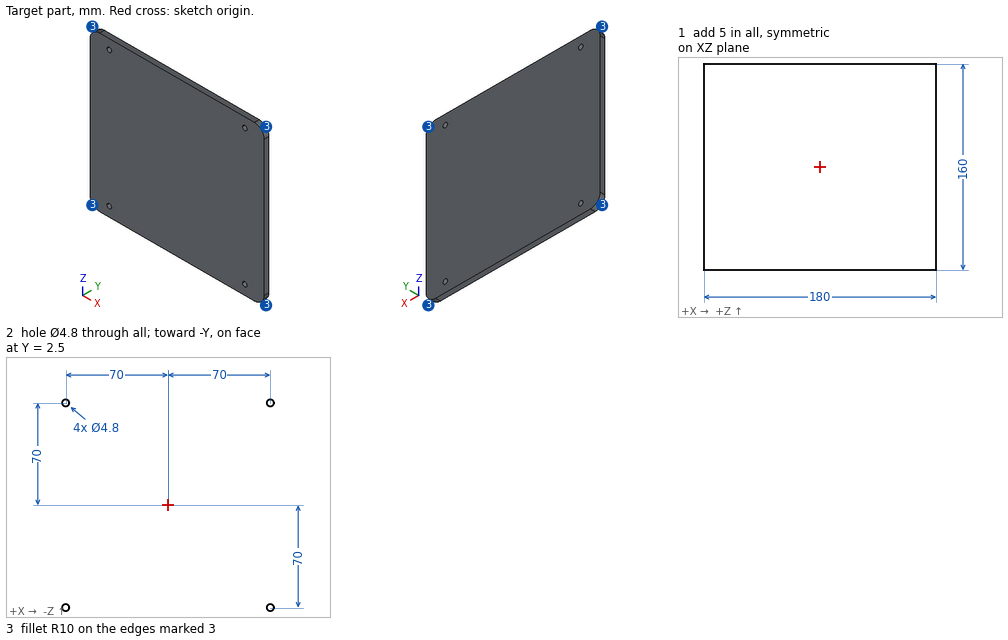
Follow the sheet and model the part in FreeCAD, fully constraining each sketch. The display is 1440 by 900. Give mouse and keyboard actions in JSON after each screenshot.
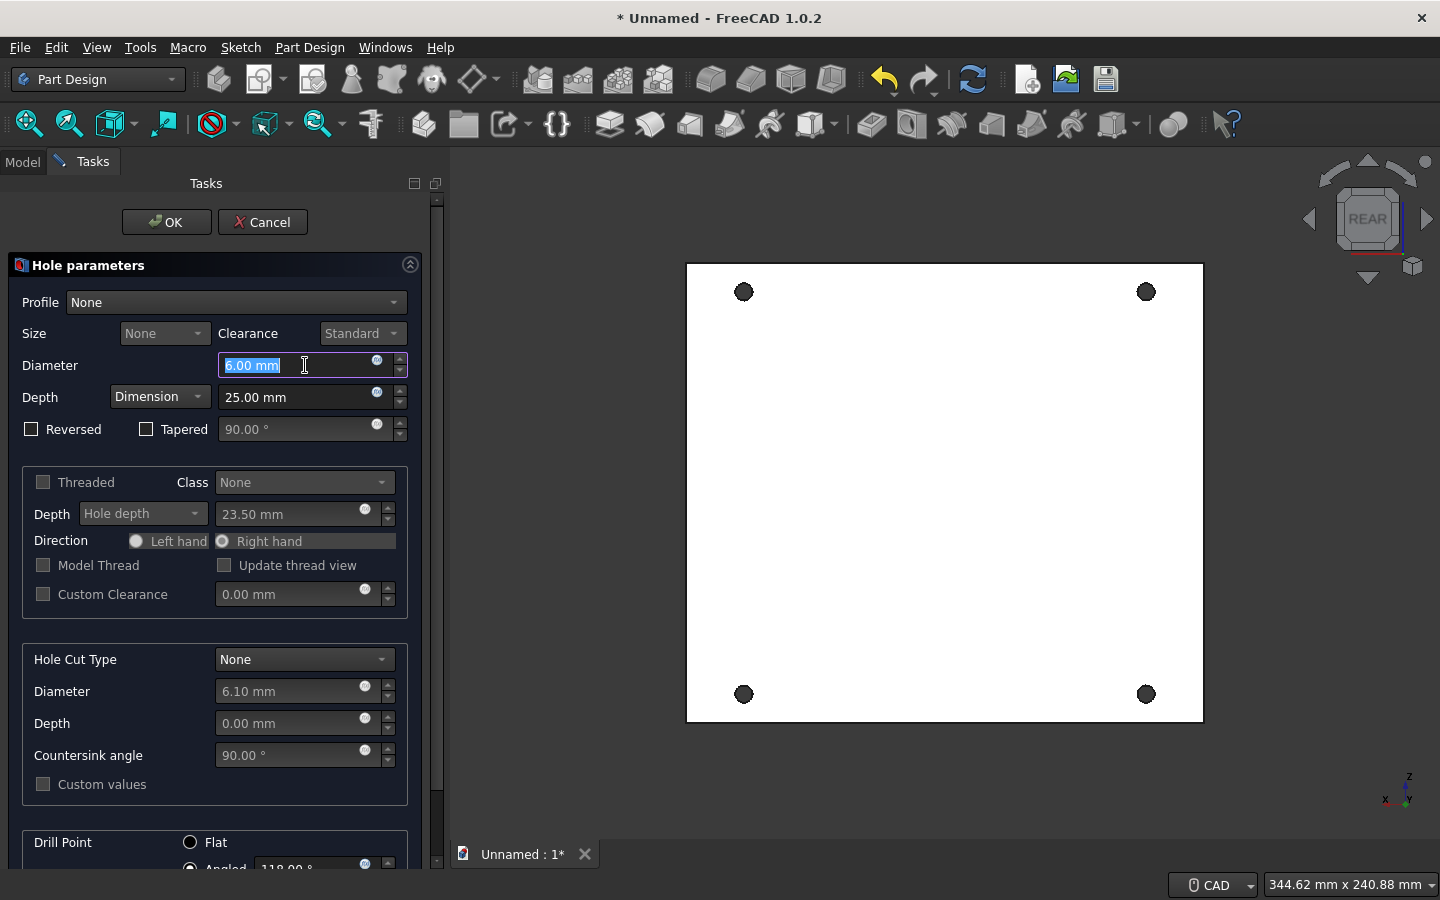
{"action": "type", "text": "4.8"}
{"action": "key", "text": "Tab"}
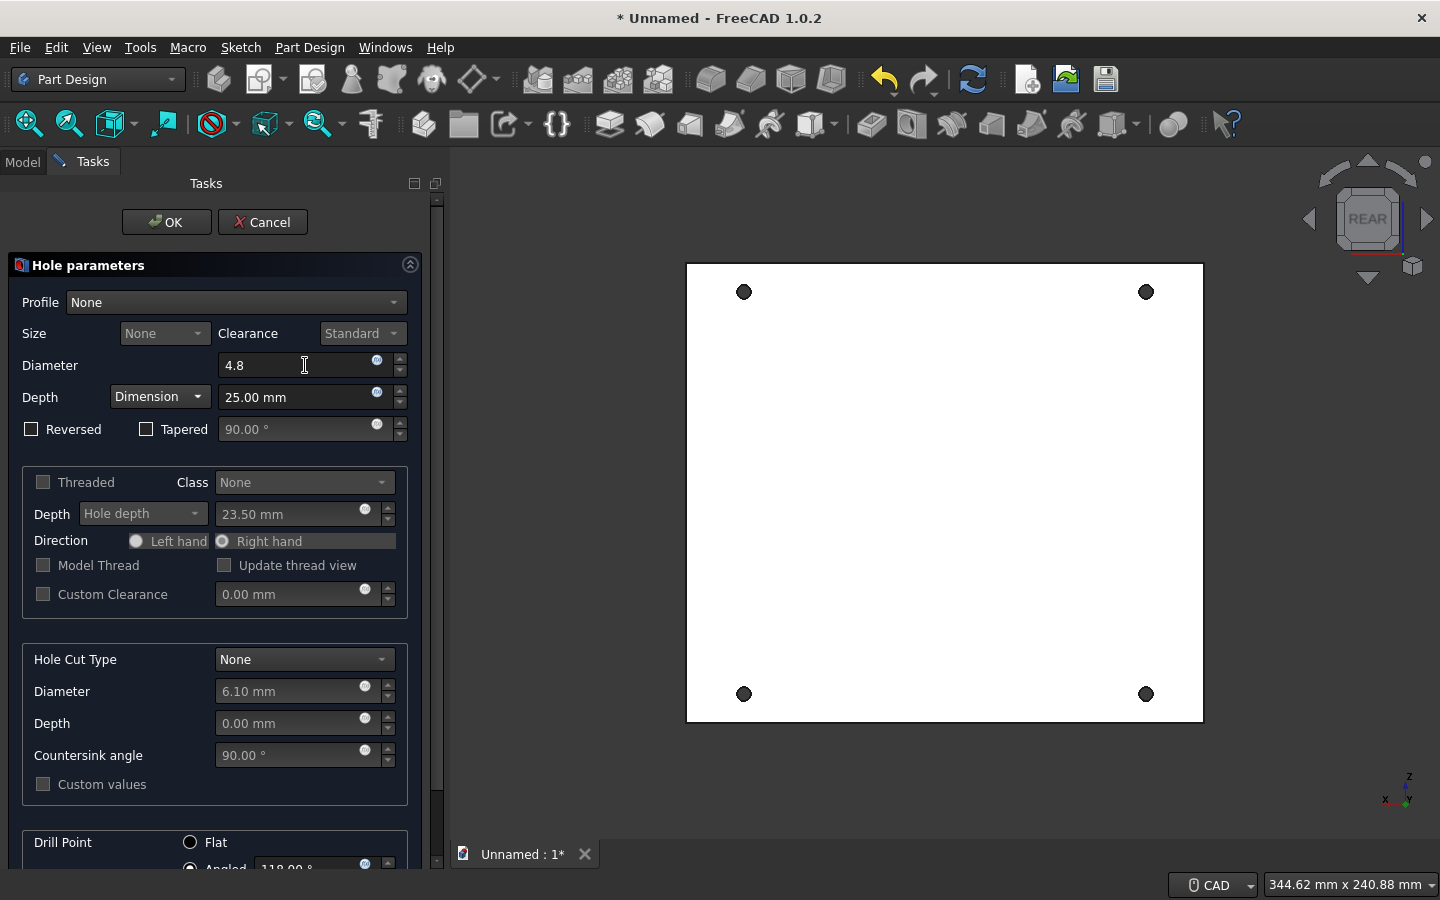
{"action": "left_click", "coordinate": [161, 396]}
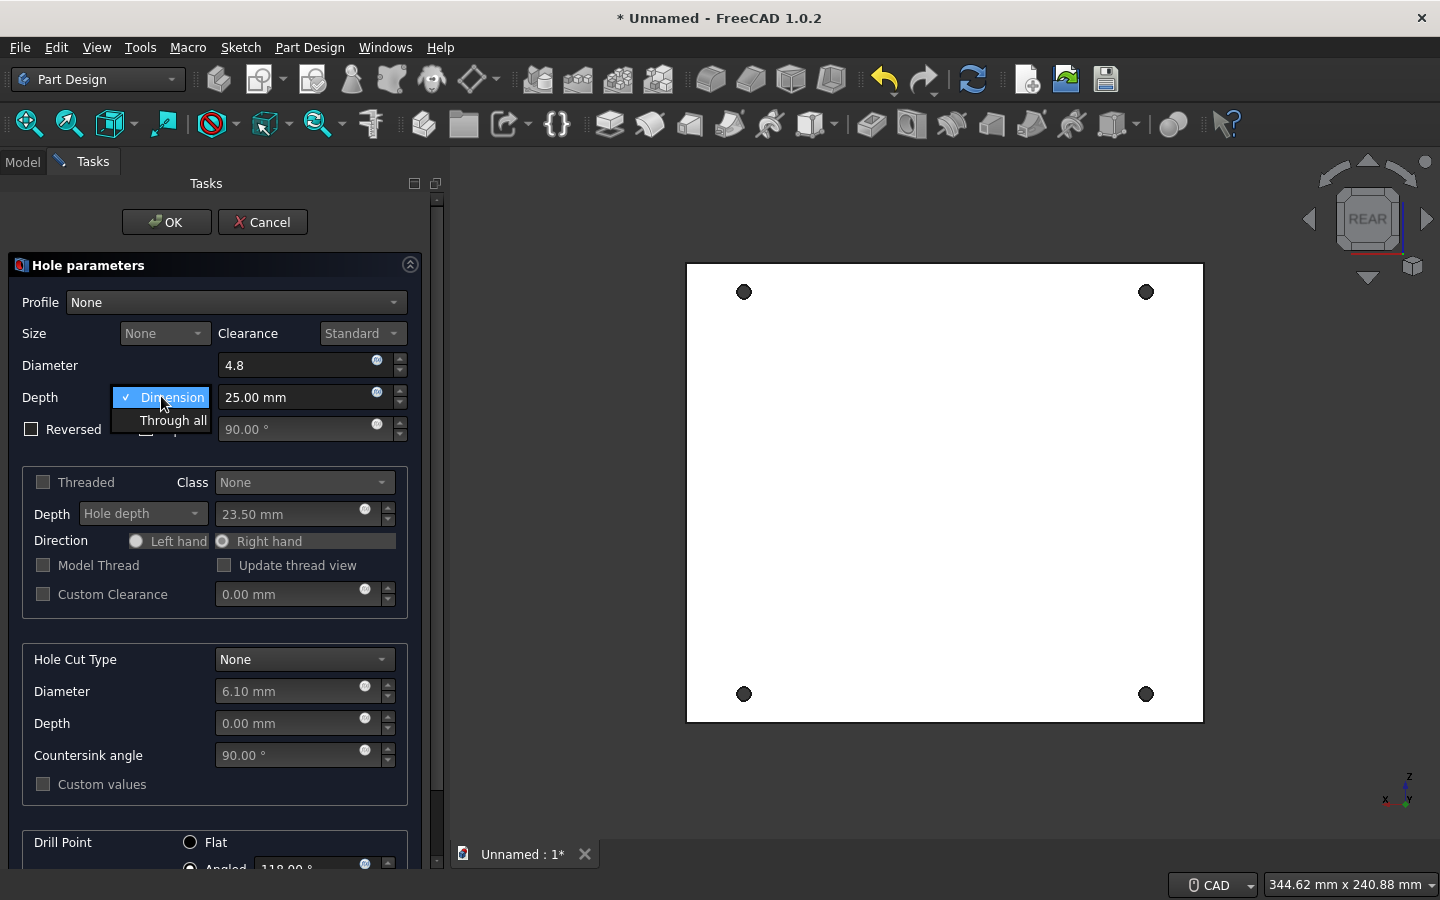
{"action": "left_click", "coordinate": [160, 420]}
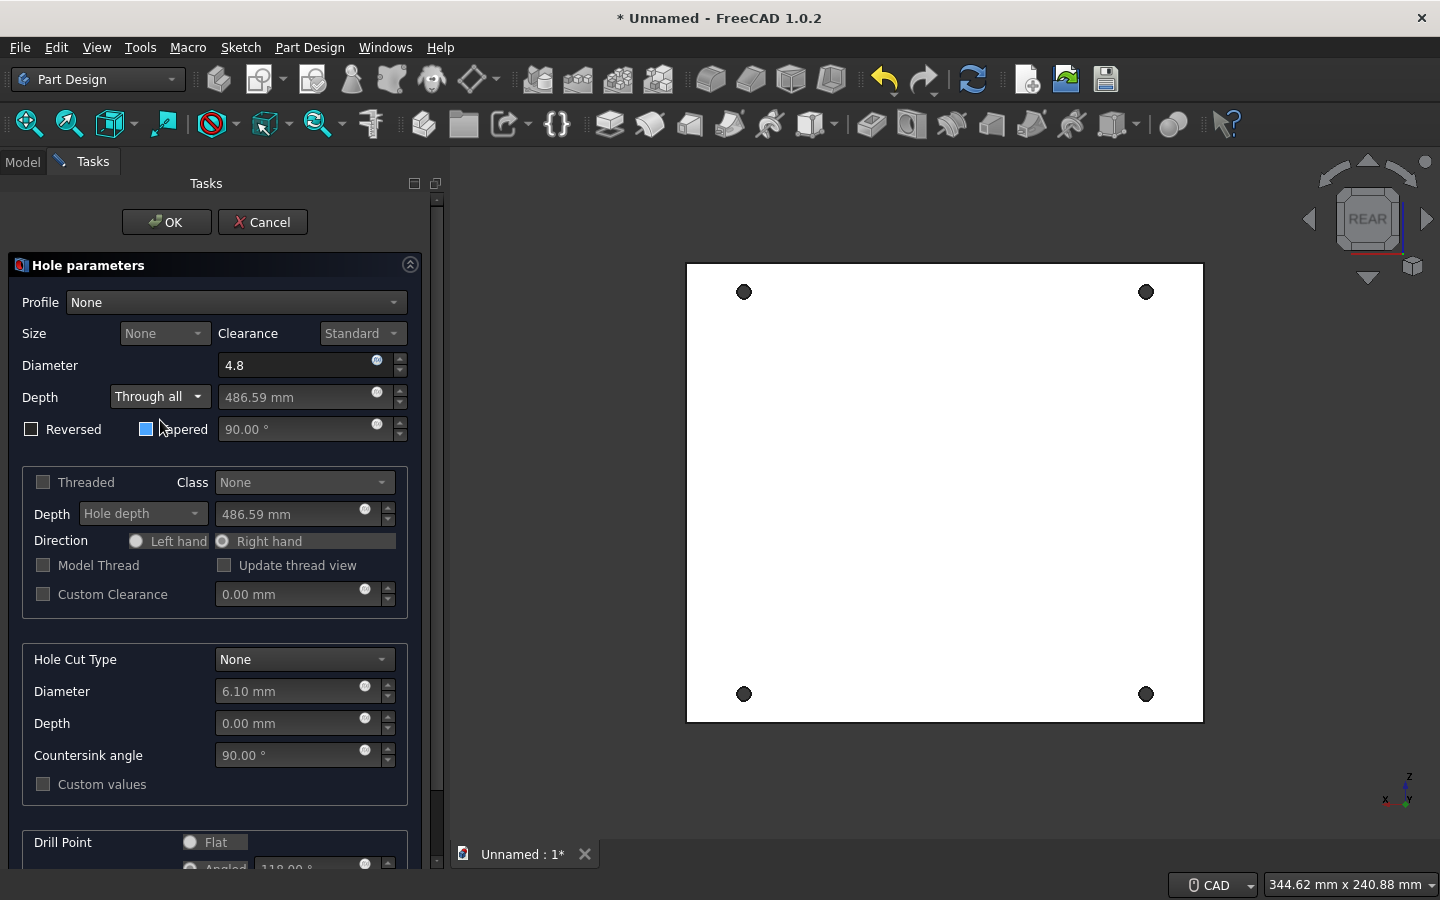
{"action": "left_click", "coordinate": [167, 222]}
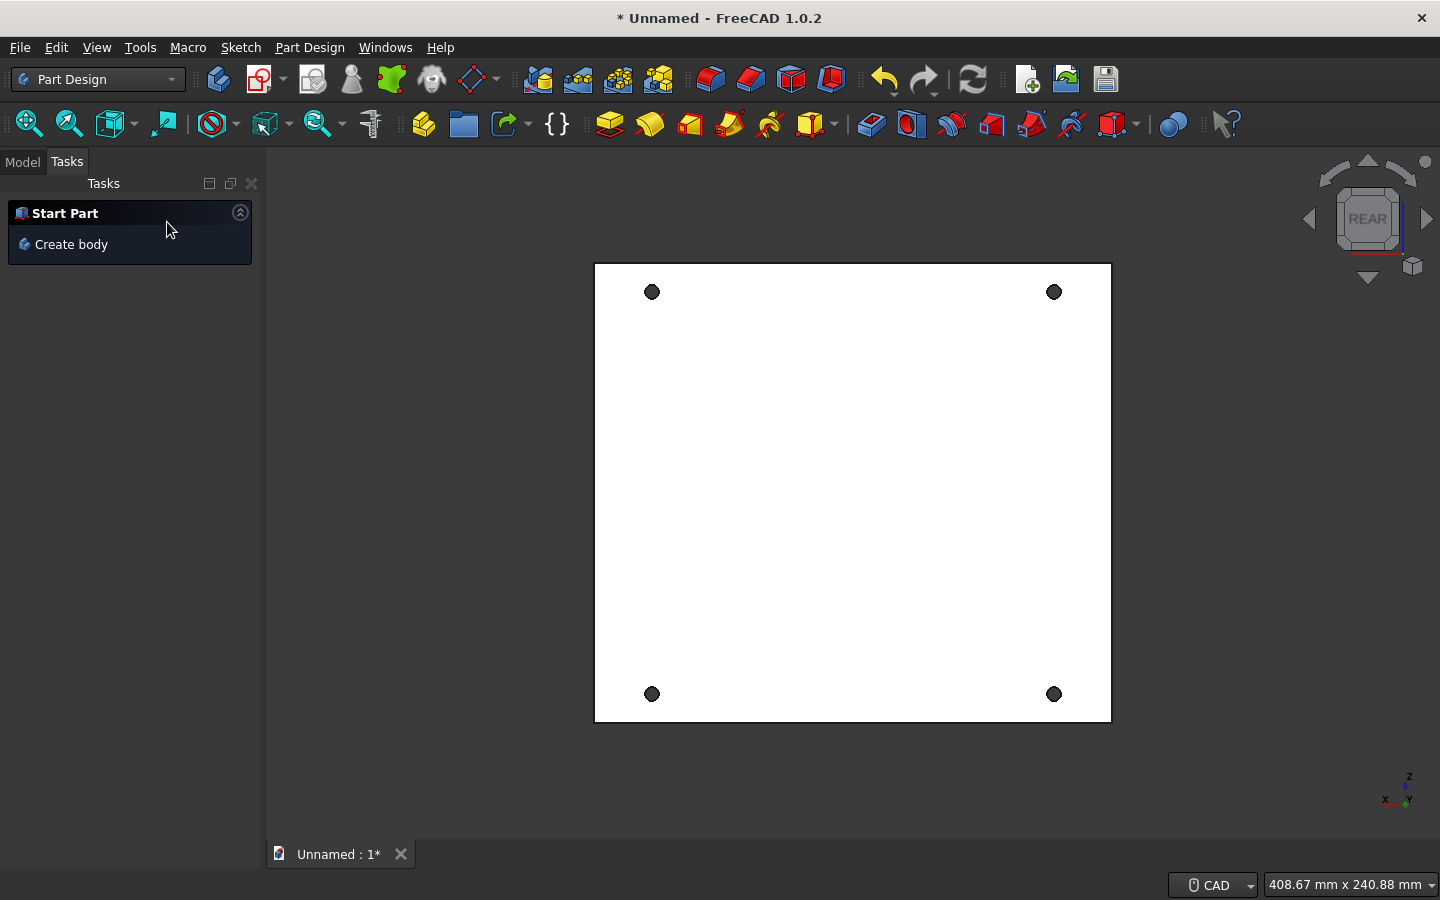
{"action": "scroll", "coordinate": [594, 262], "scroll_direction": "up", "scroll_amount": 6}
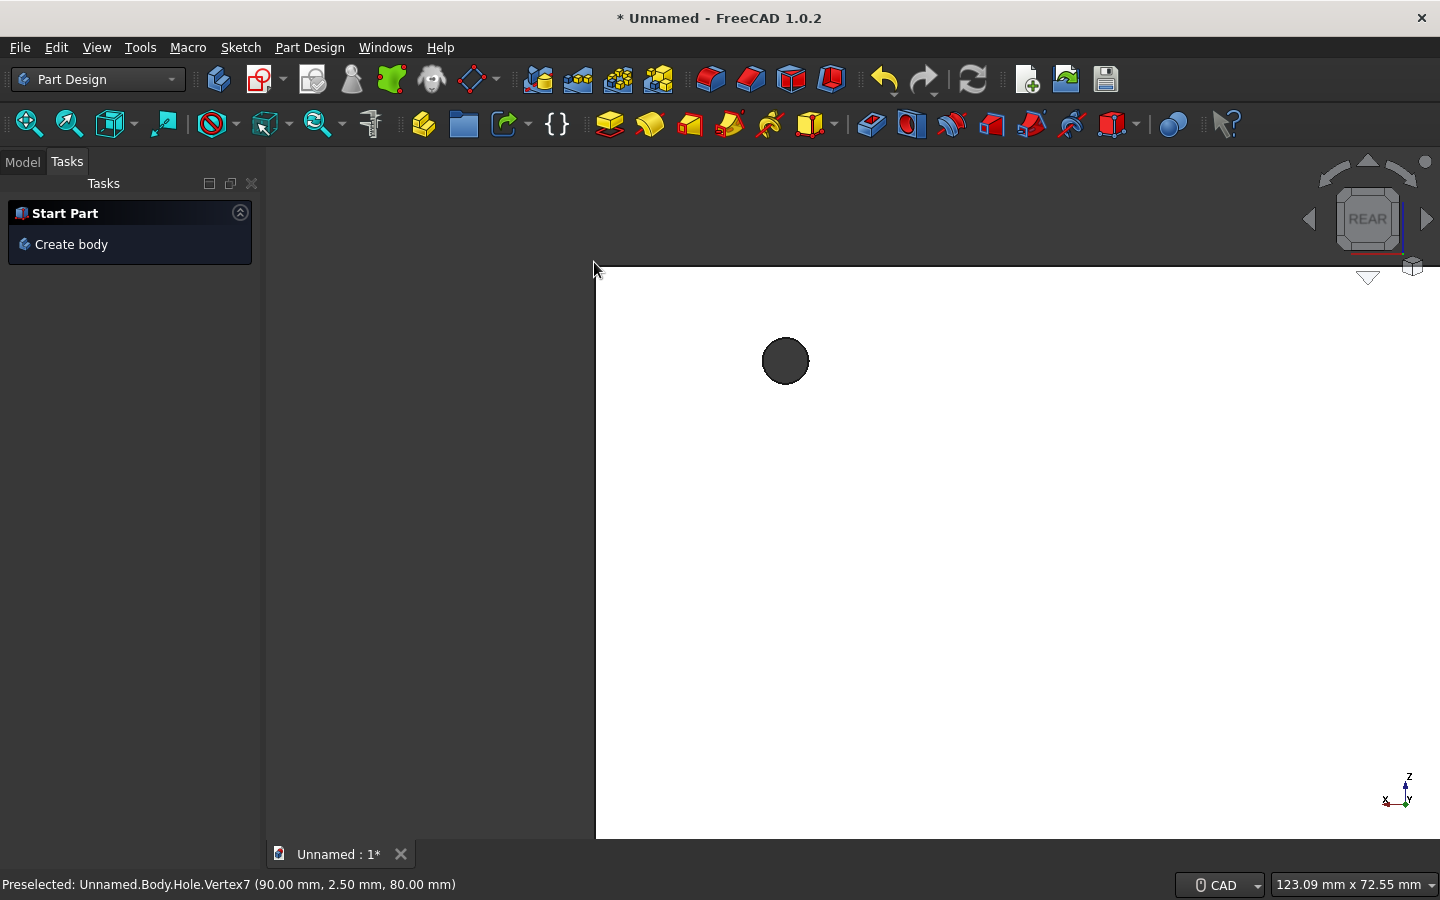
{"action": "left_click", "coordinate": [30, 124]}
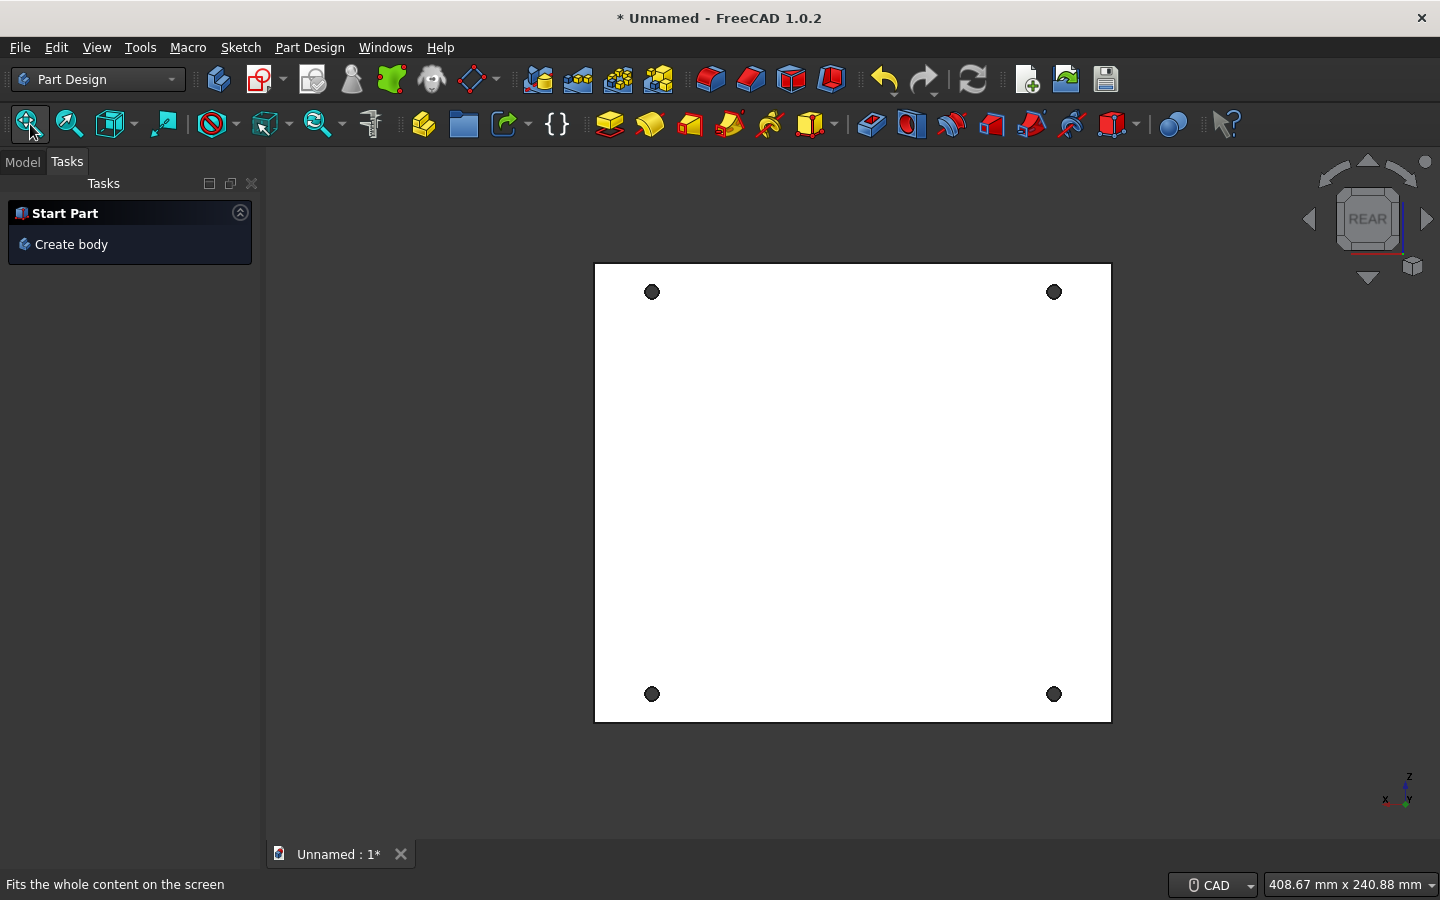
{"action": "key", "text": "0"}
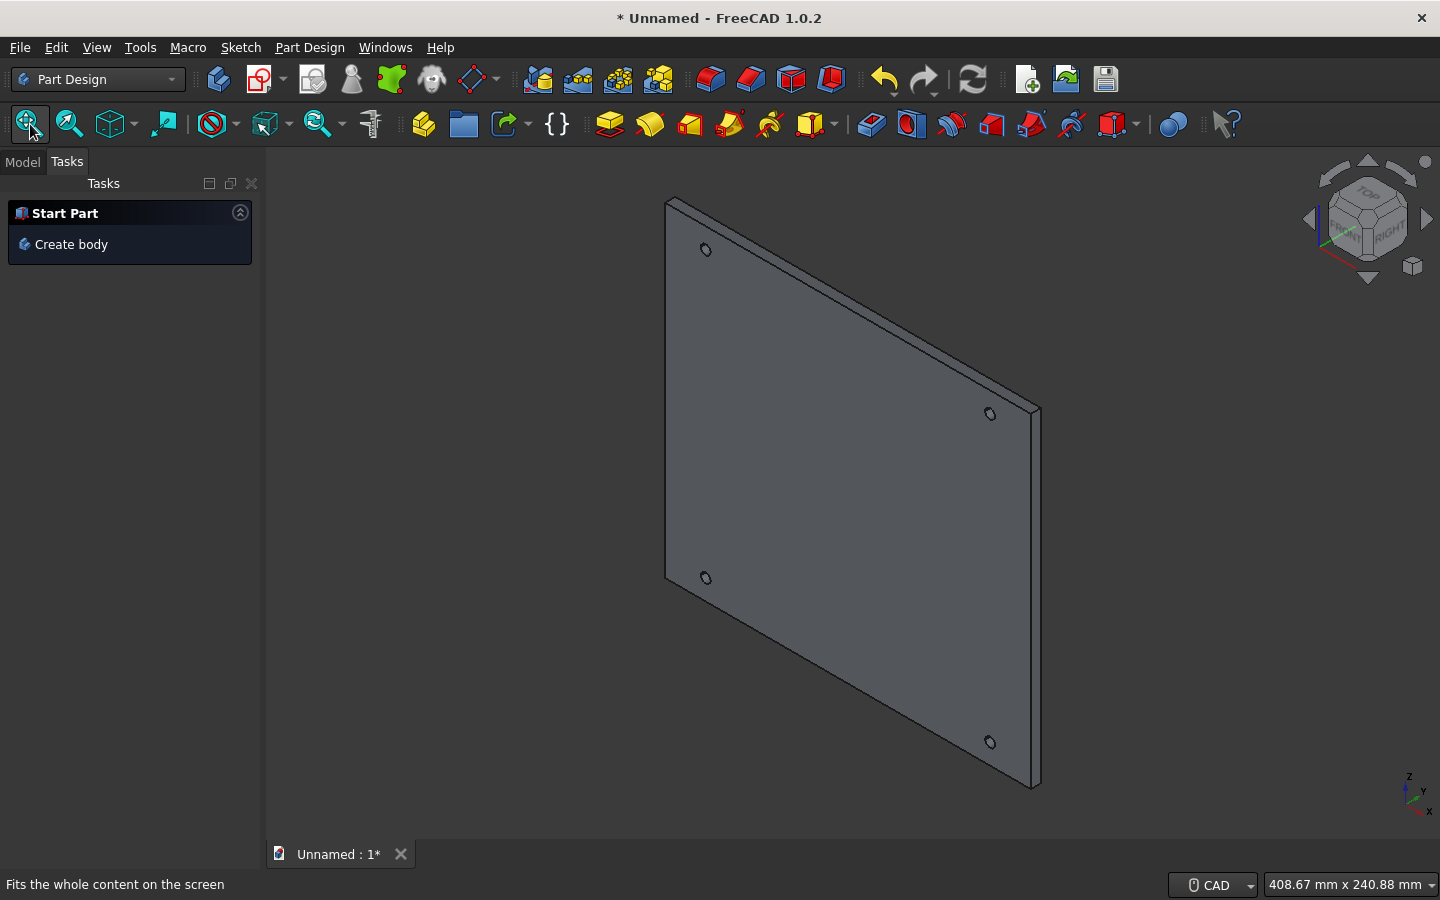
{"action": "left_click", "coordinate": [1037, 409]}